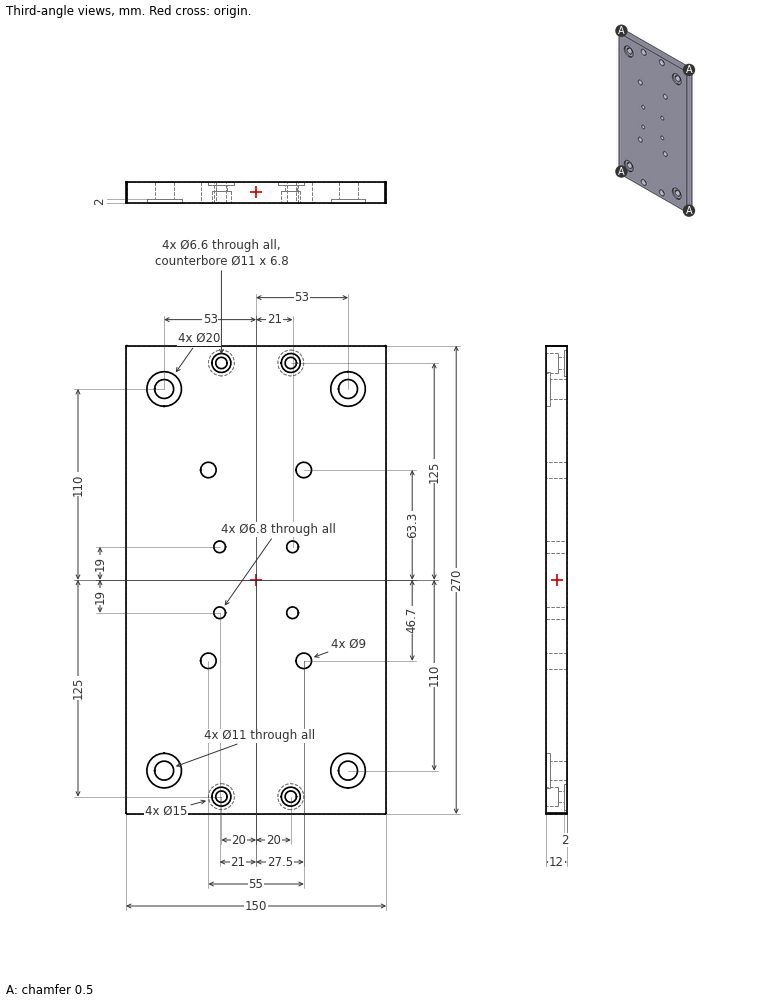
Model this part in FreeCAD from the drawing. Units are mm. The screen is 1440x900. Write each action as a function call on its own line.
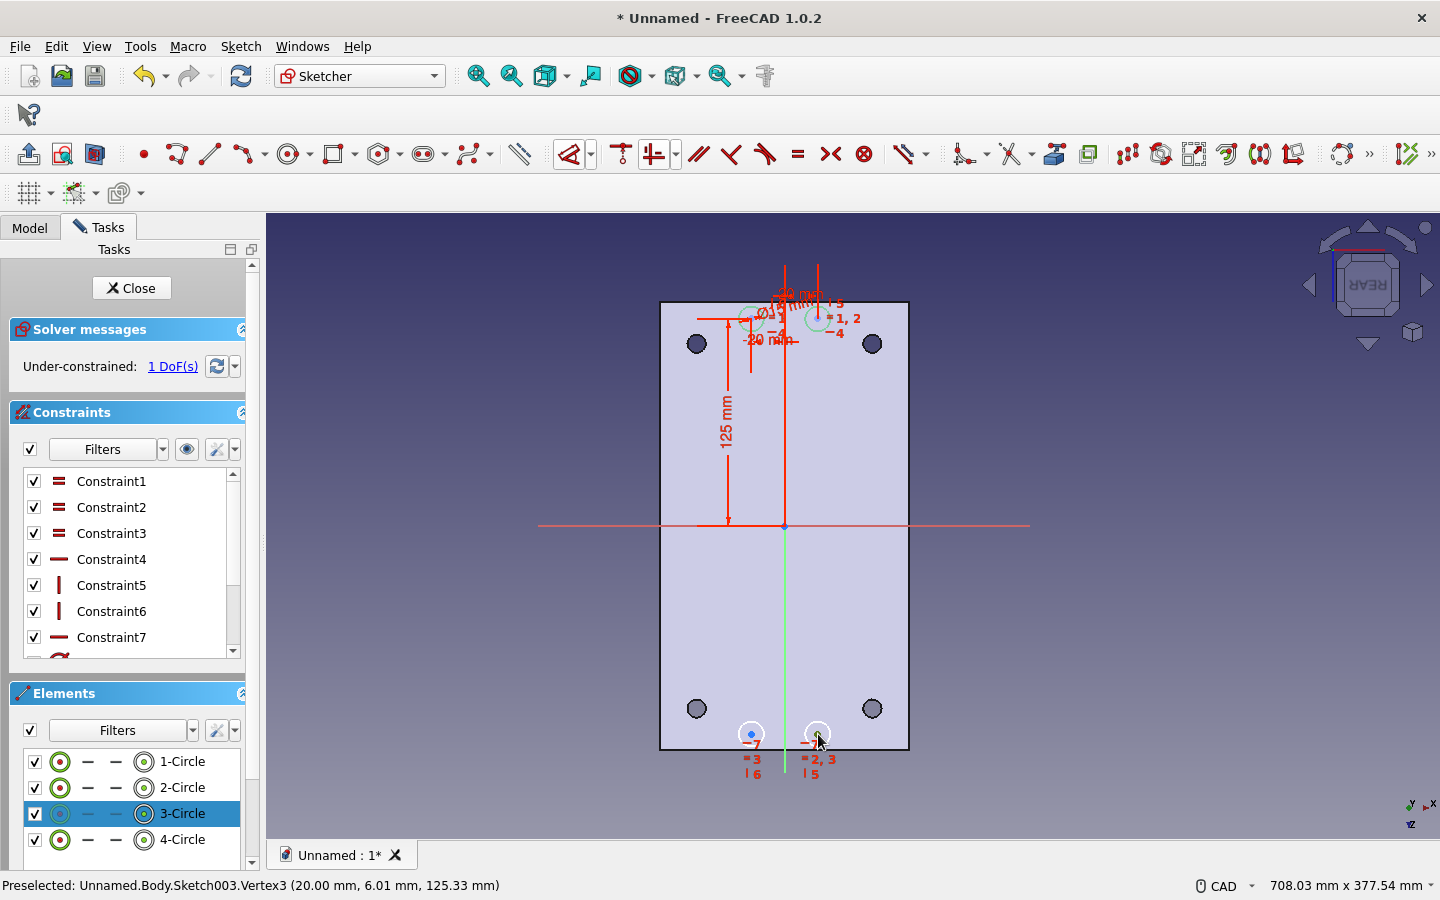
key(i)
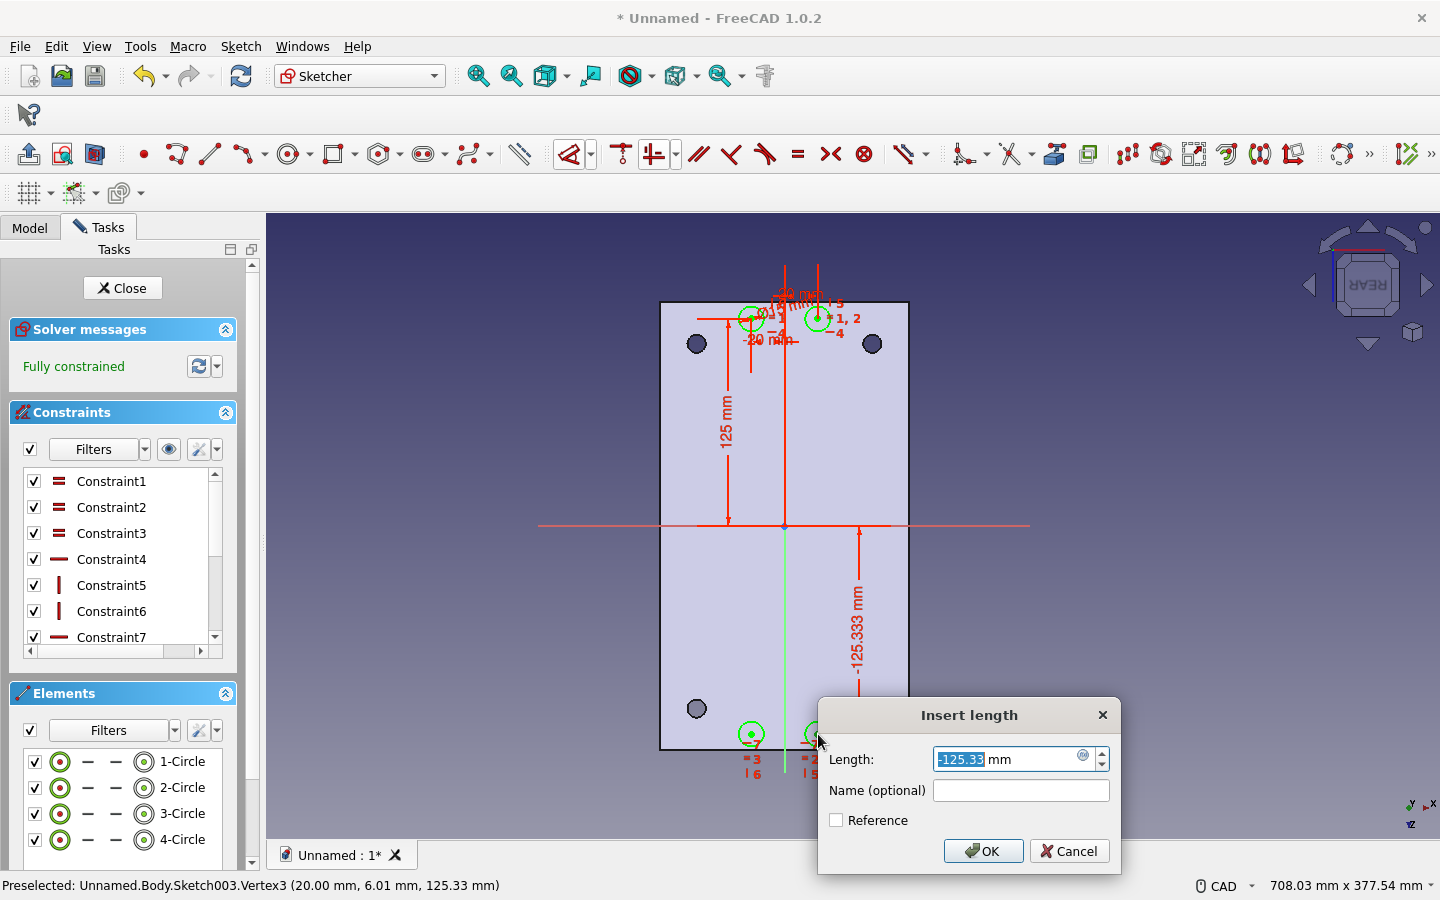
text(-125)
key(Return)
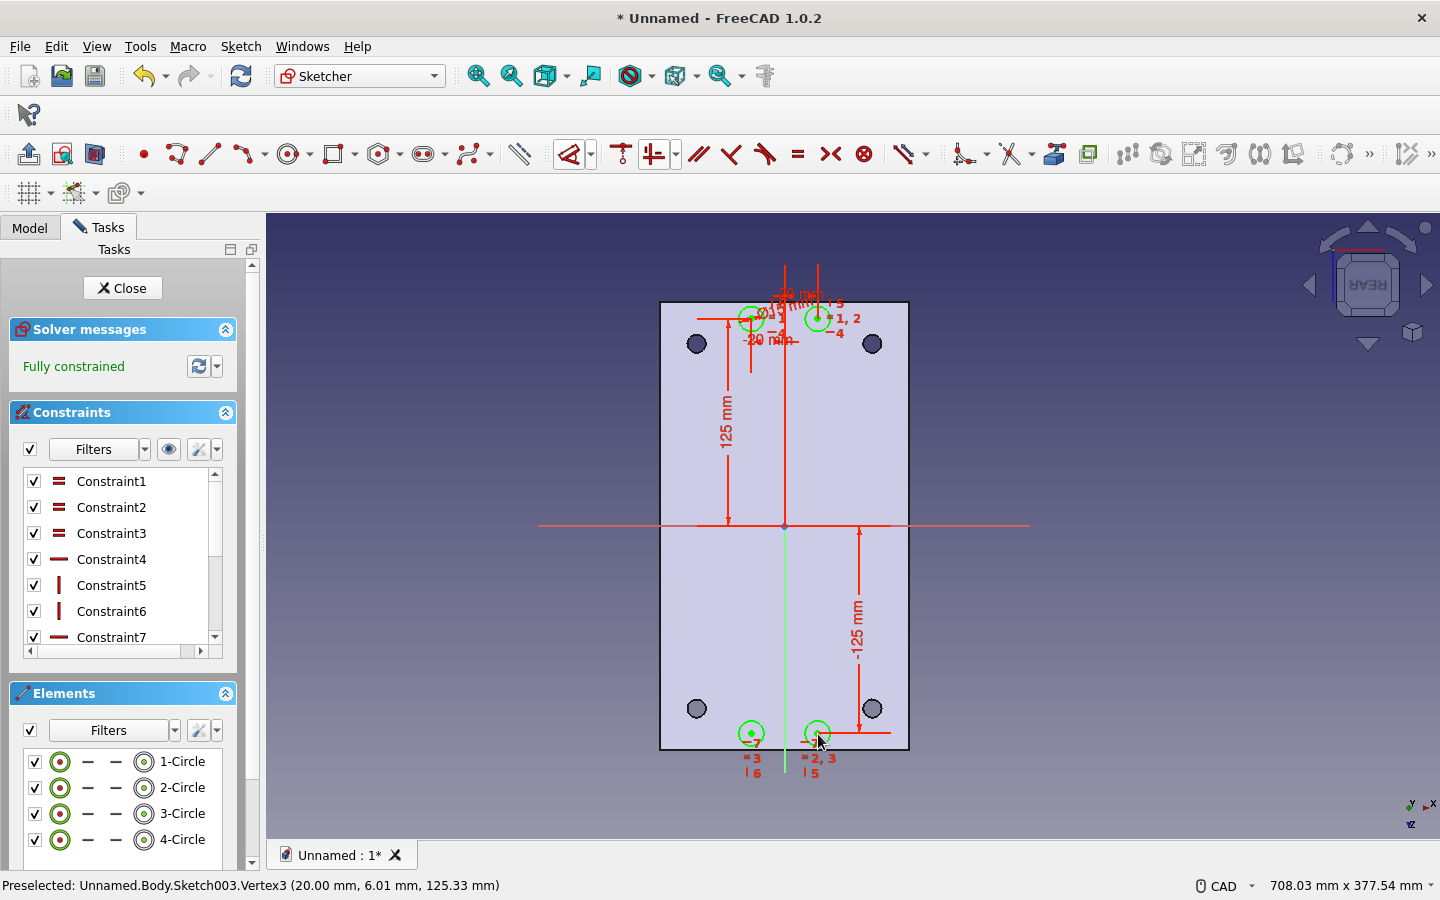
click(123, 288)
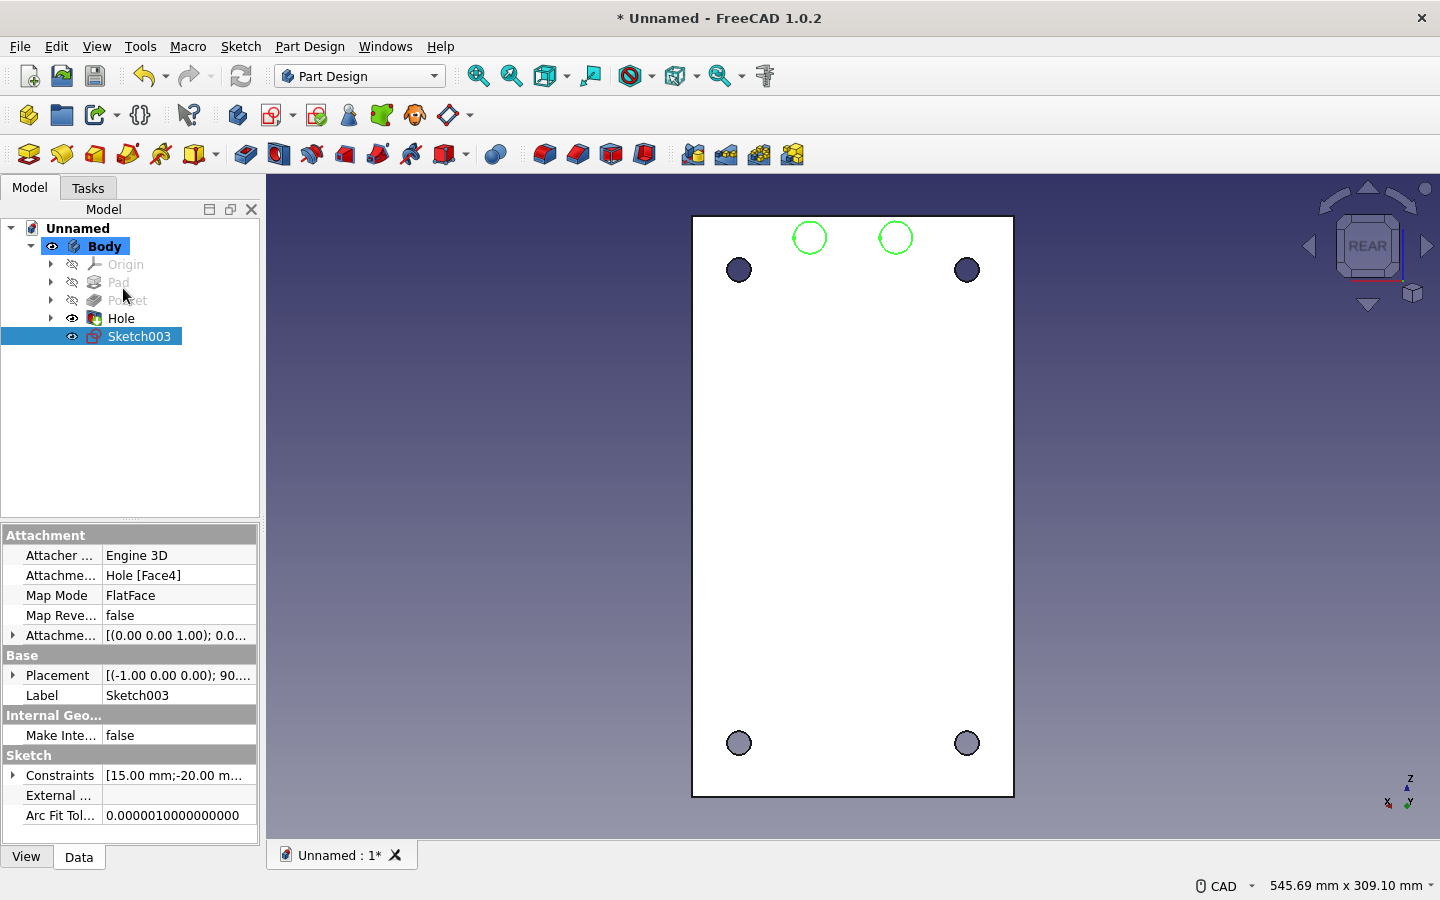
click(246, 154)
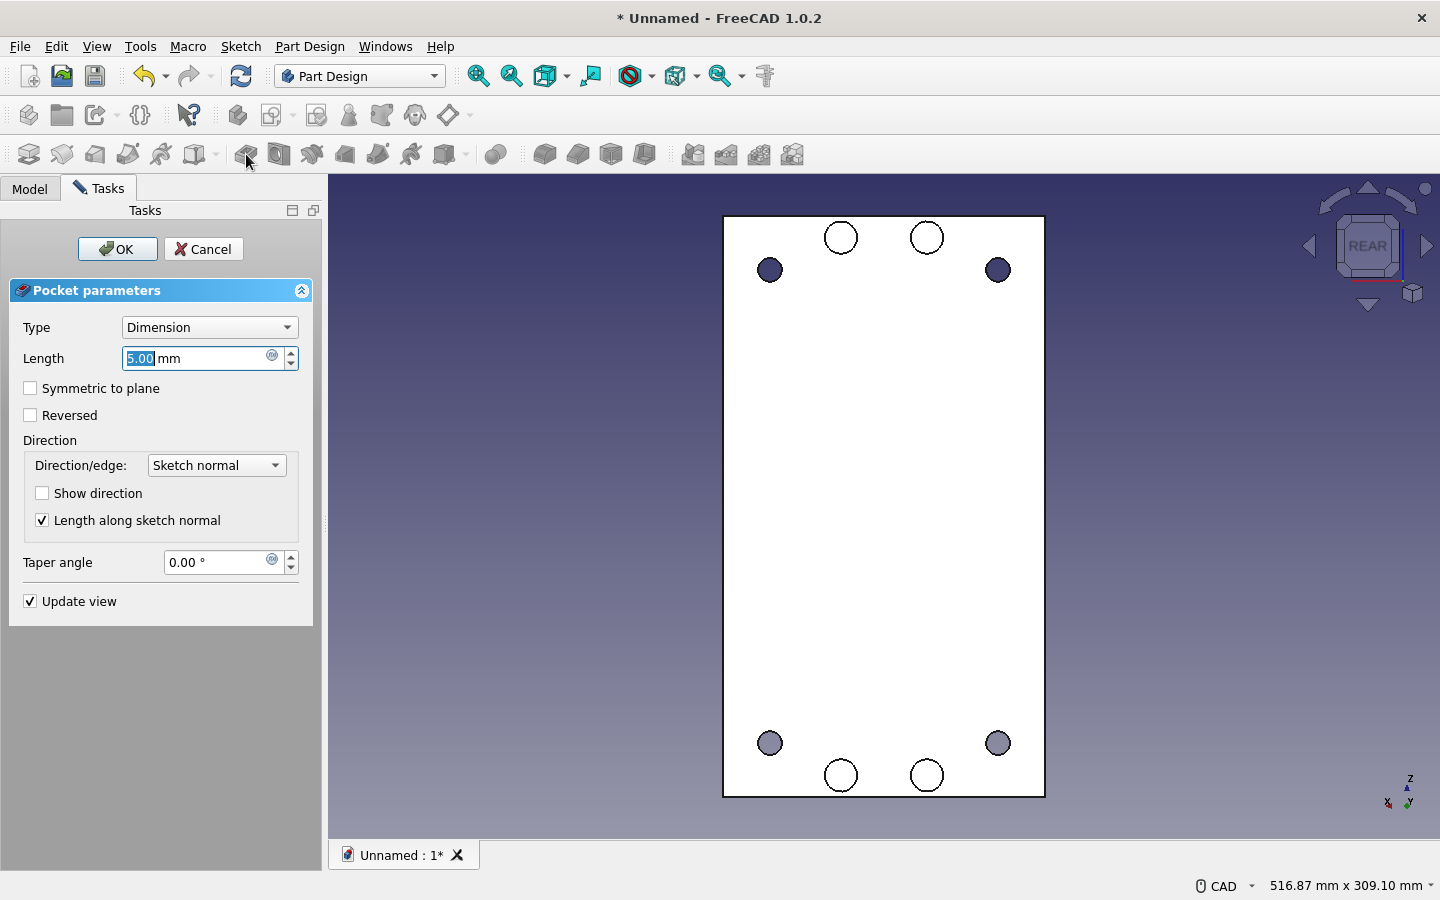
text(2)
key(Tab)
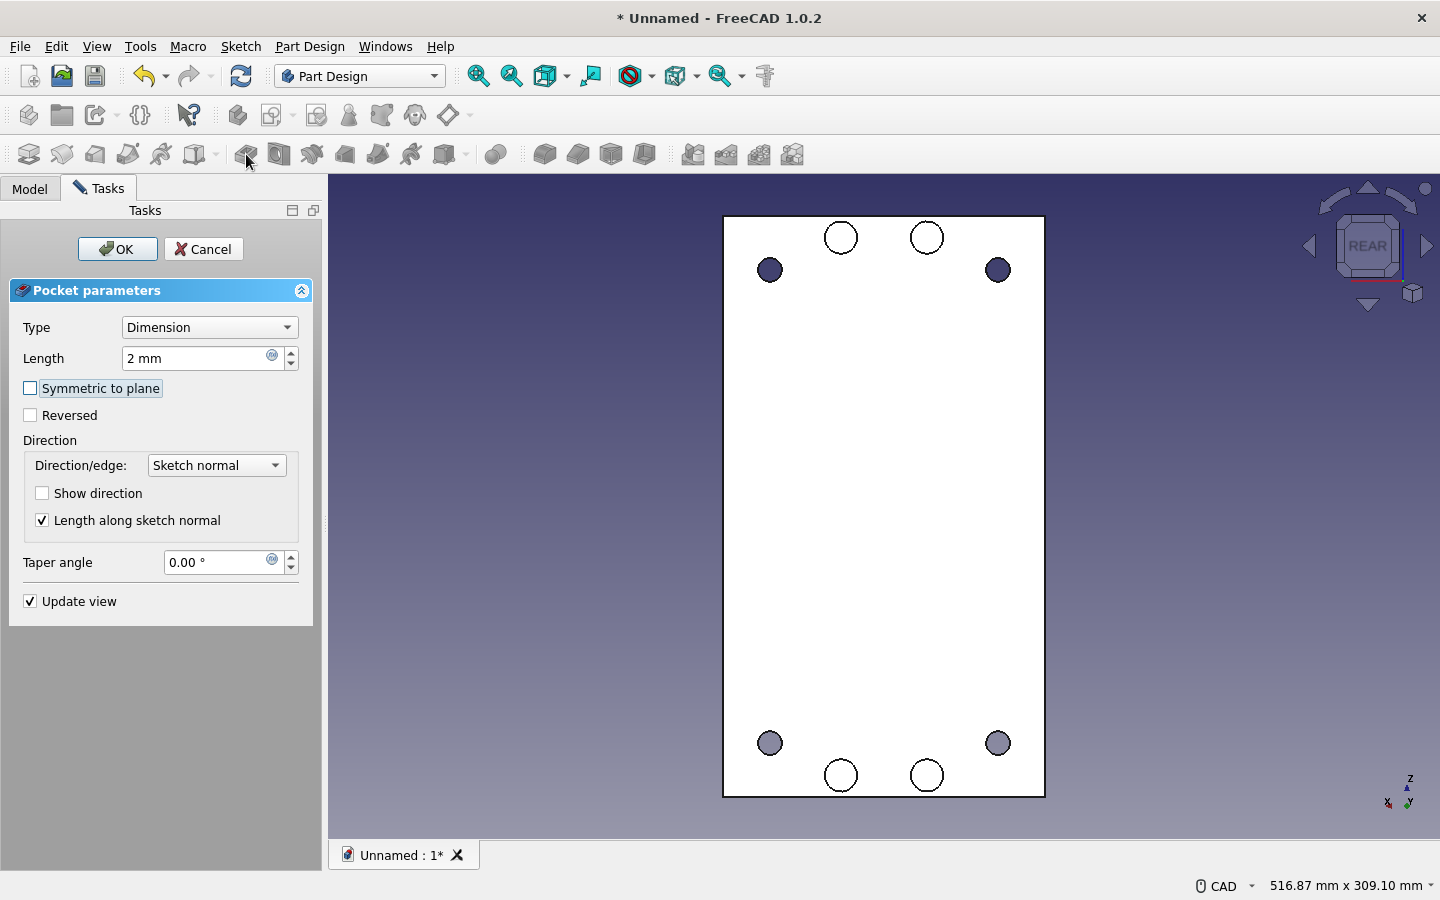
click(118, 249)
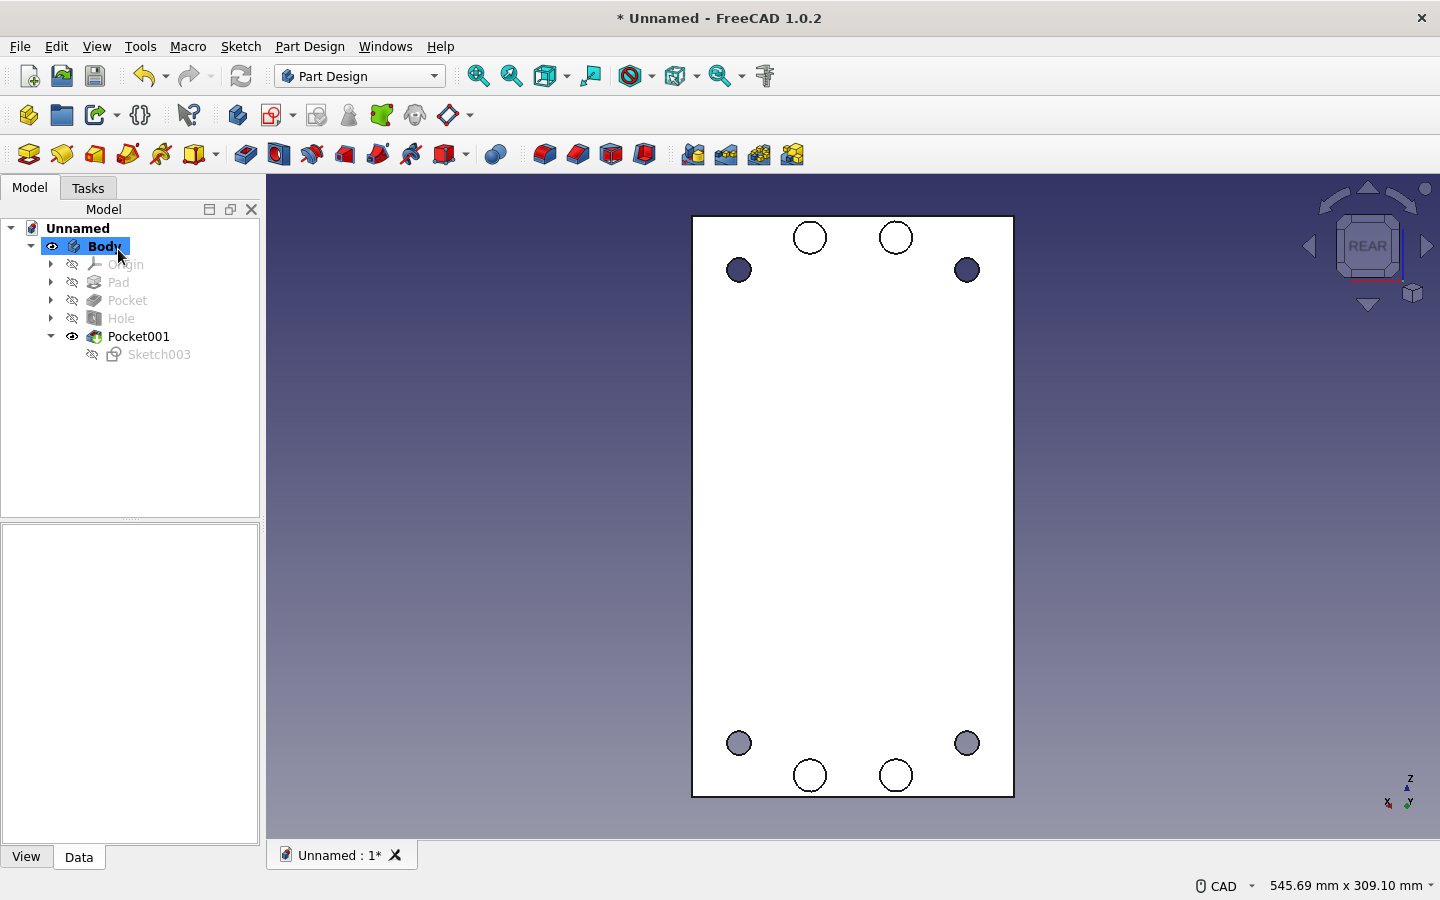
key(0)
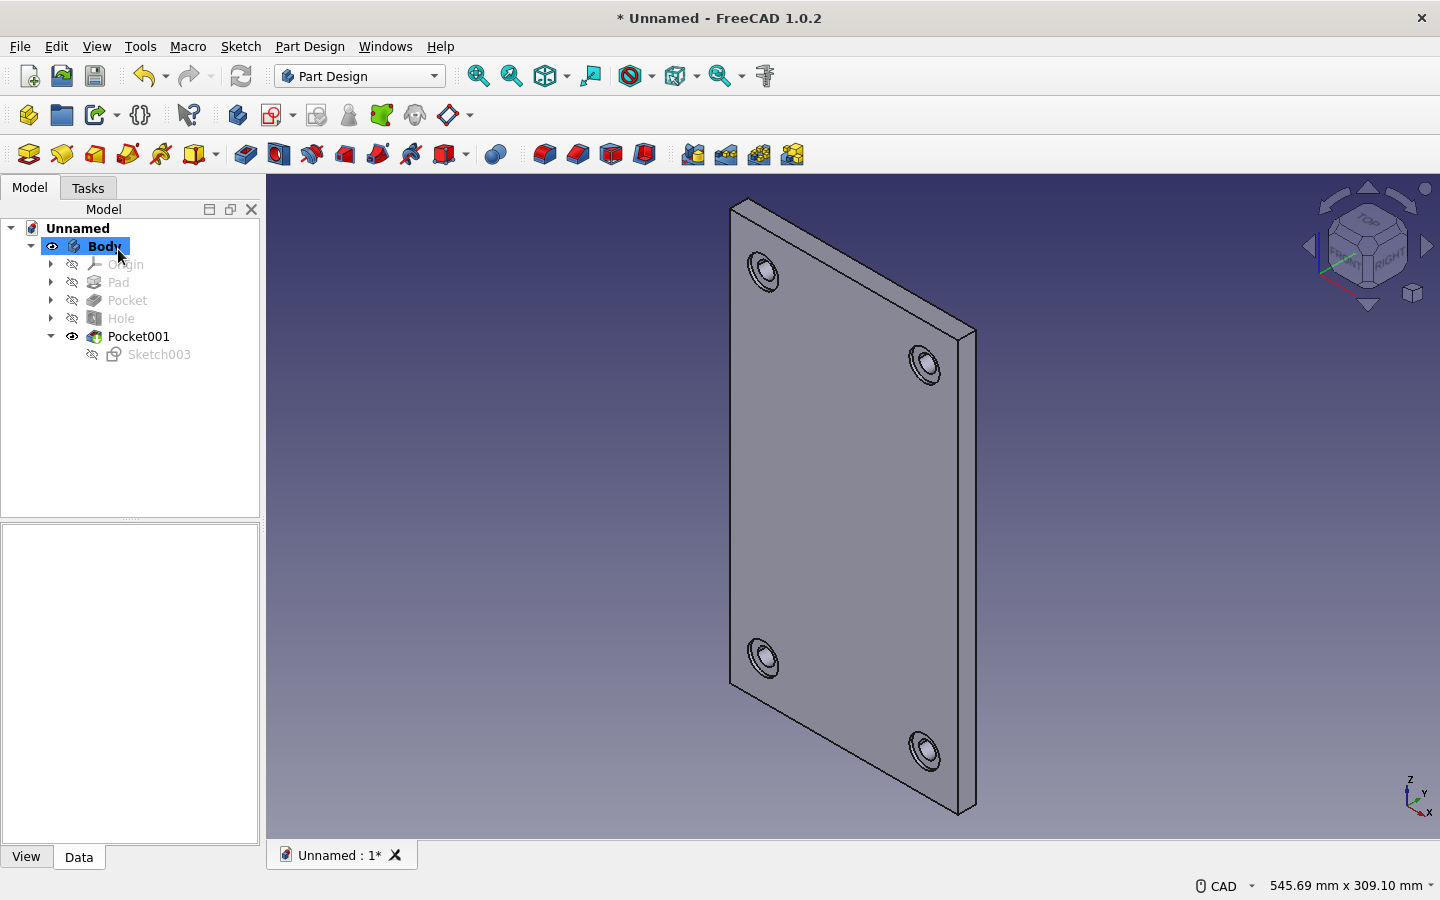
click(844, 443)